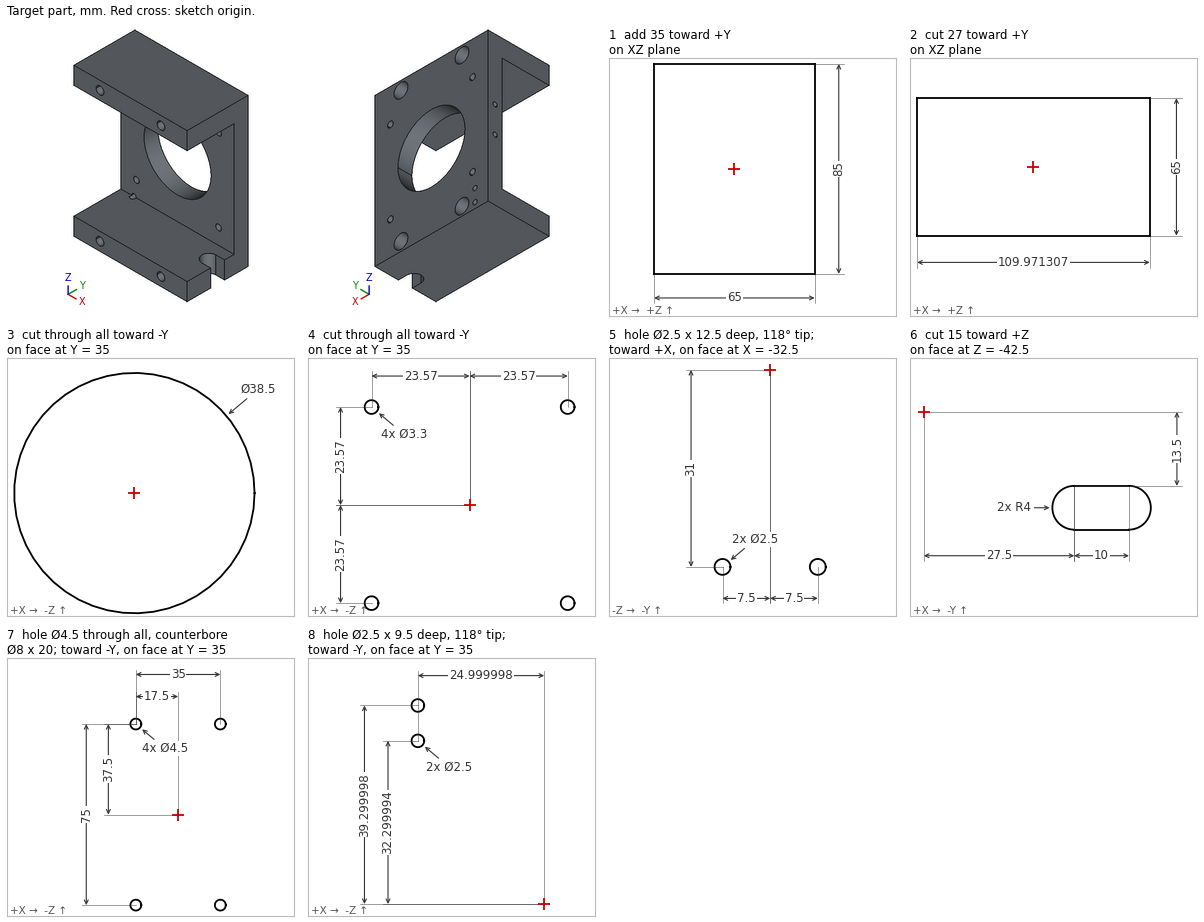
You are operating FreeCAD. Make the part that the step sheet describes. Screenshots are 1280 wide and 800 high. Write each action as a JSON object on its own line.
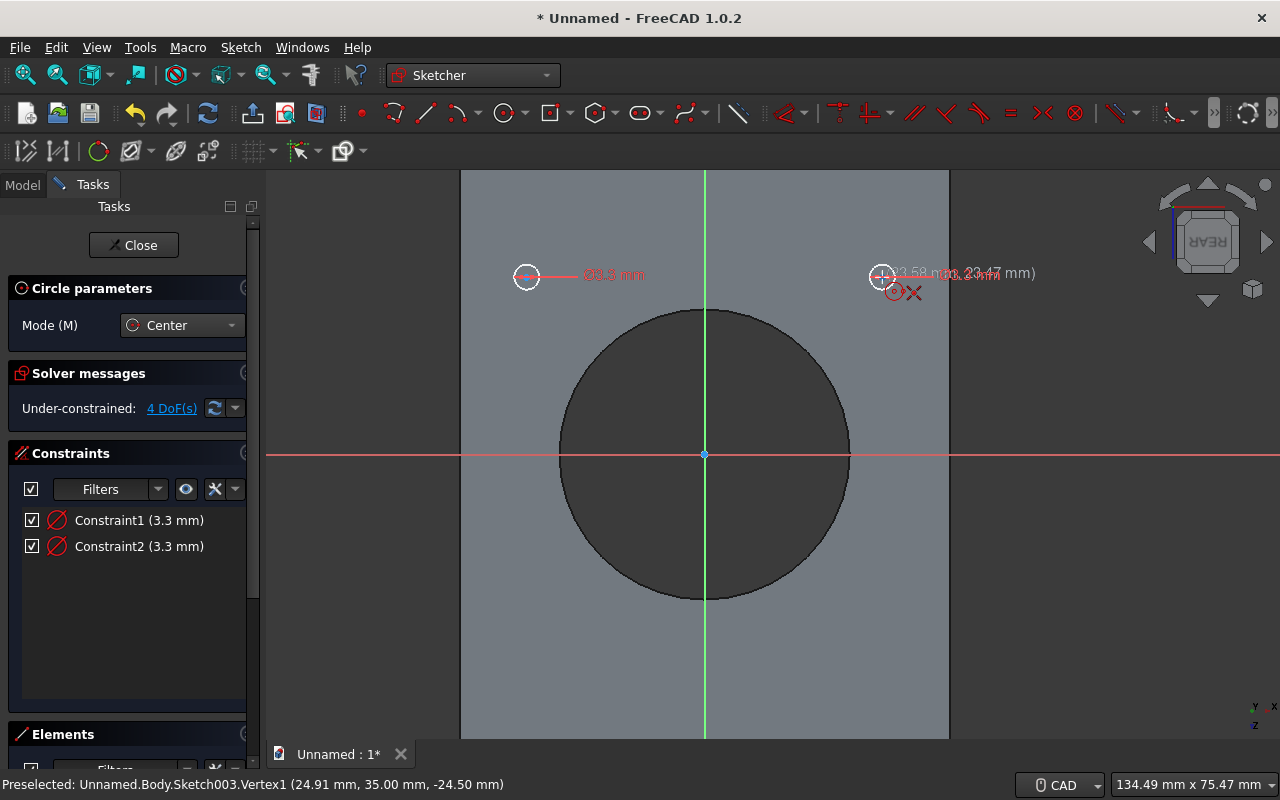
{"action": "scroll", "coordinate": [527, 632], "scroll_direction": "up", "scroll_amount": 4}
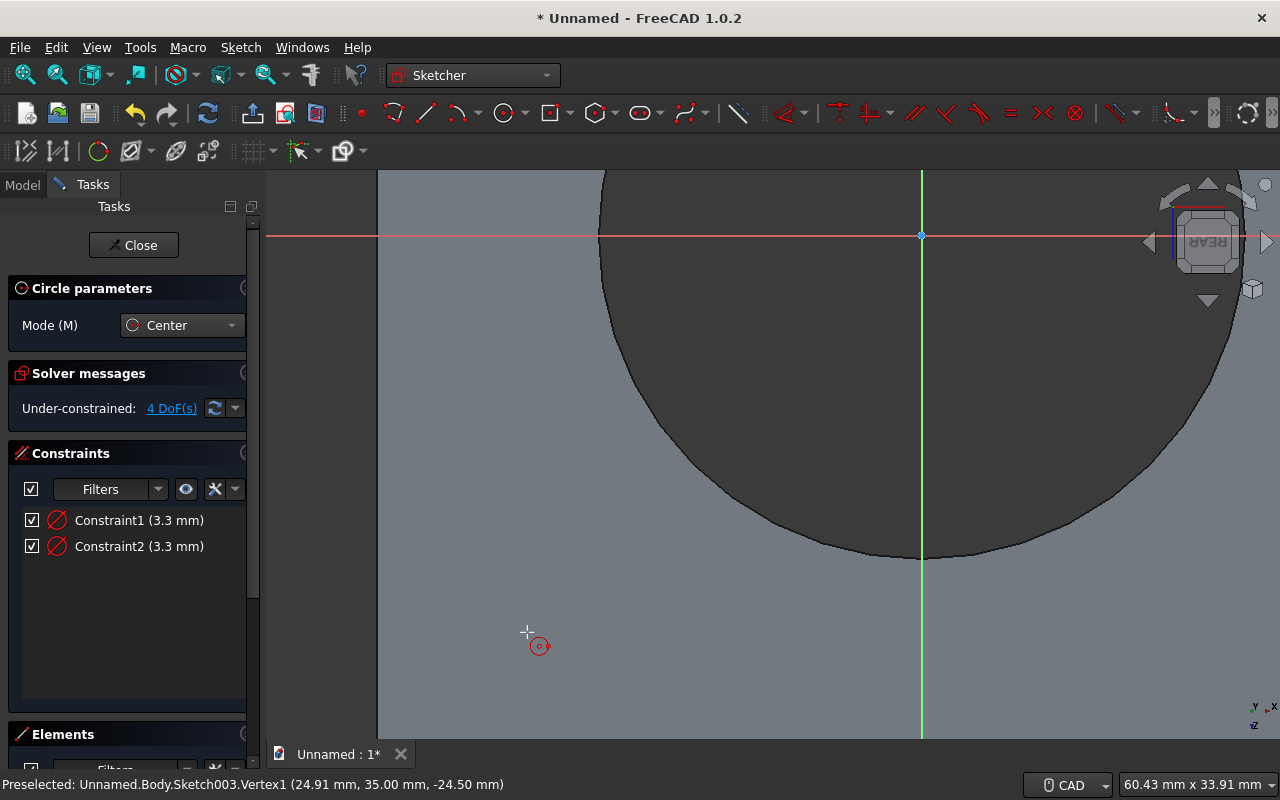
{"action": "left_click", "coordinate": [526, 631]}
{"action": "mouse_move", "coordinate": [546, 612]}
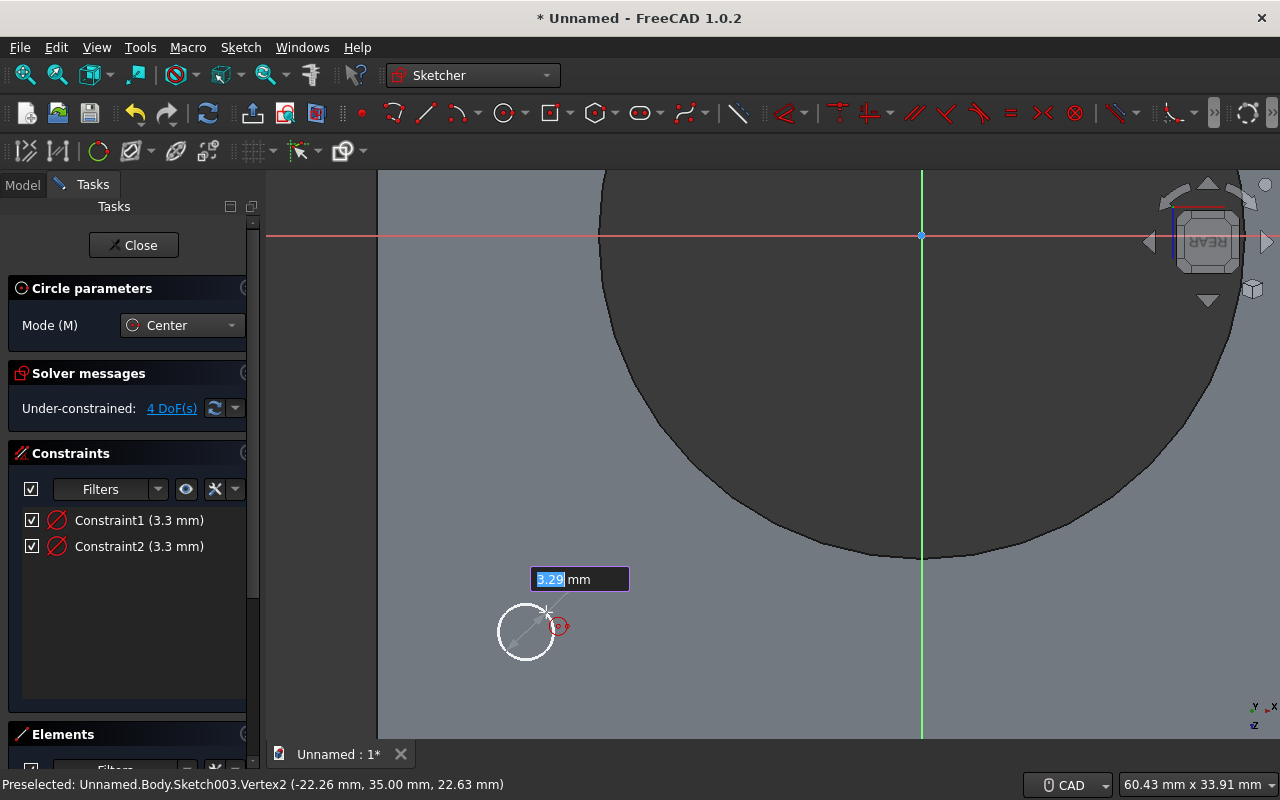
{"action": "type", "text": "3.3"}
{"action": "key", "text": "Return"}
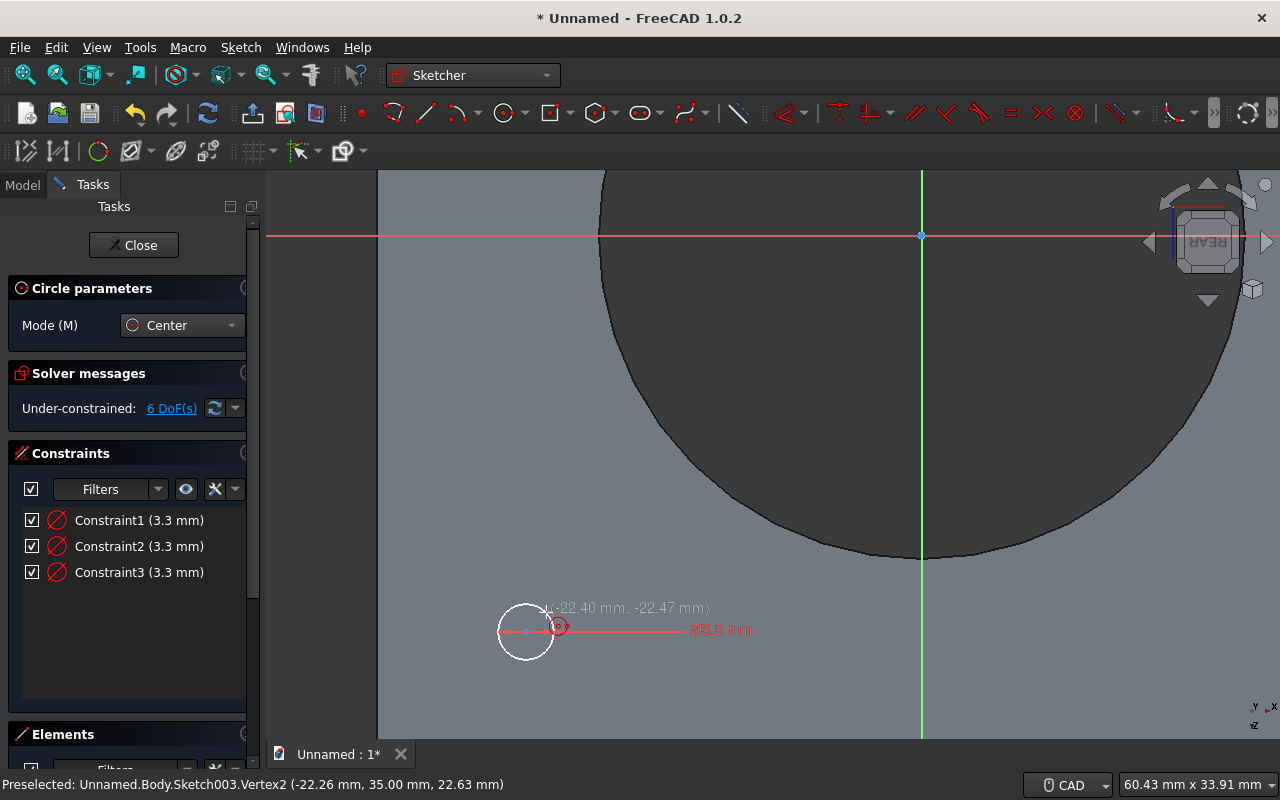
{"action": "scroll", "coordinate": [527, 633], "scroll_direction": "down", "scroll_amount": 4}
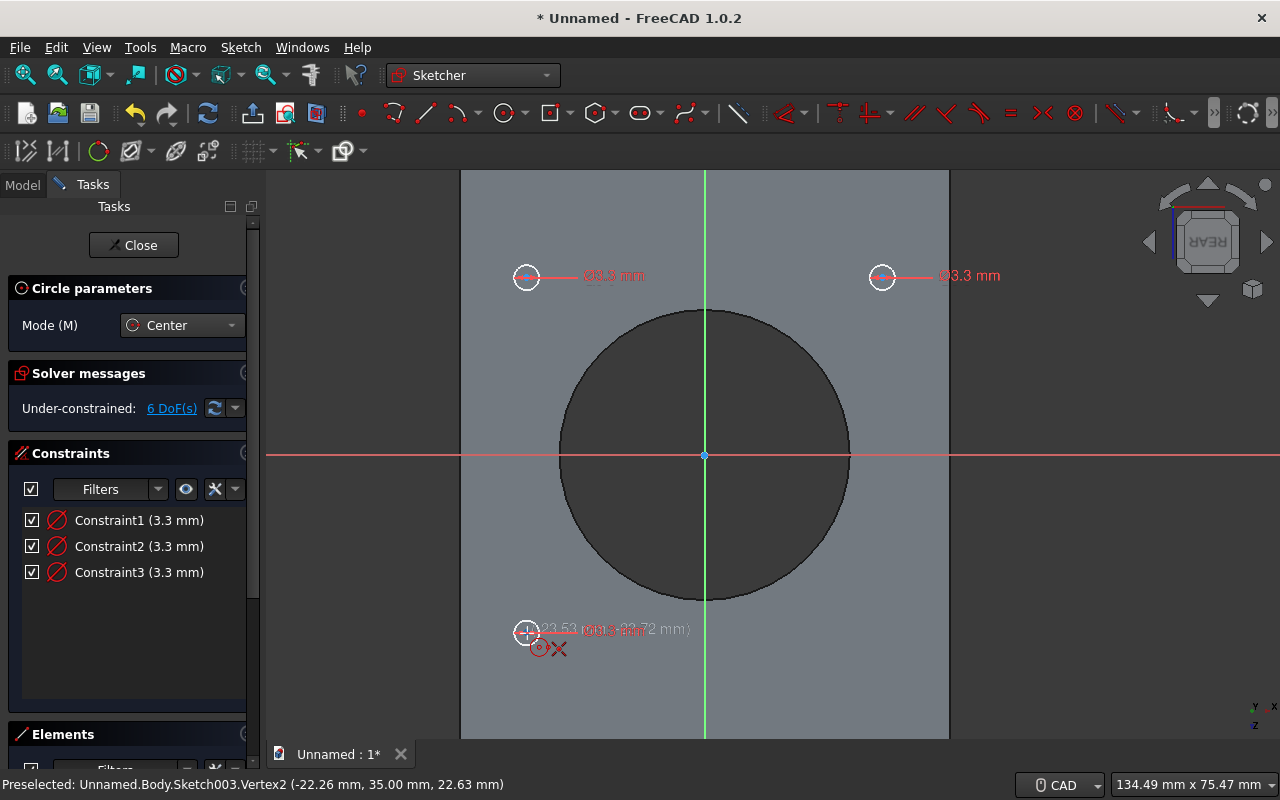
{"action": "scroll", "coordinate": [882, 633], "scroll_direction": "up", "scroll_amount": 4}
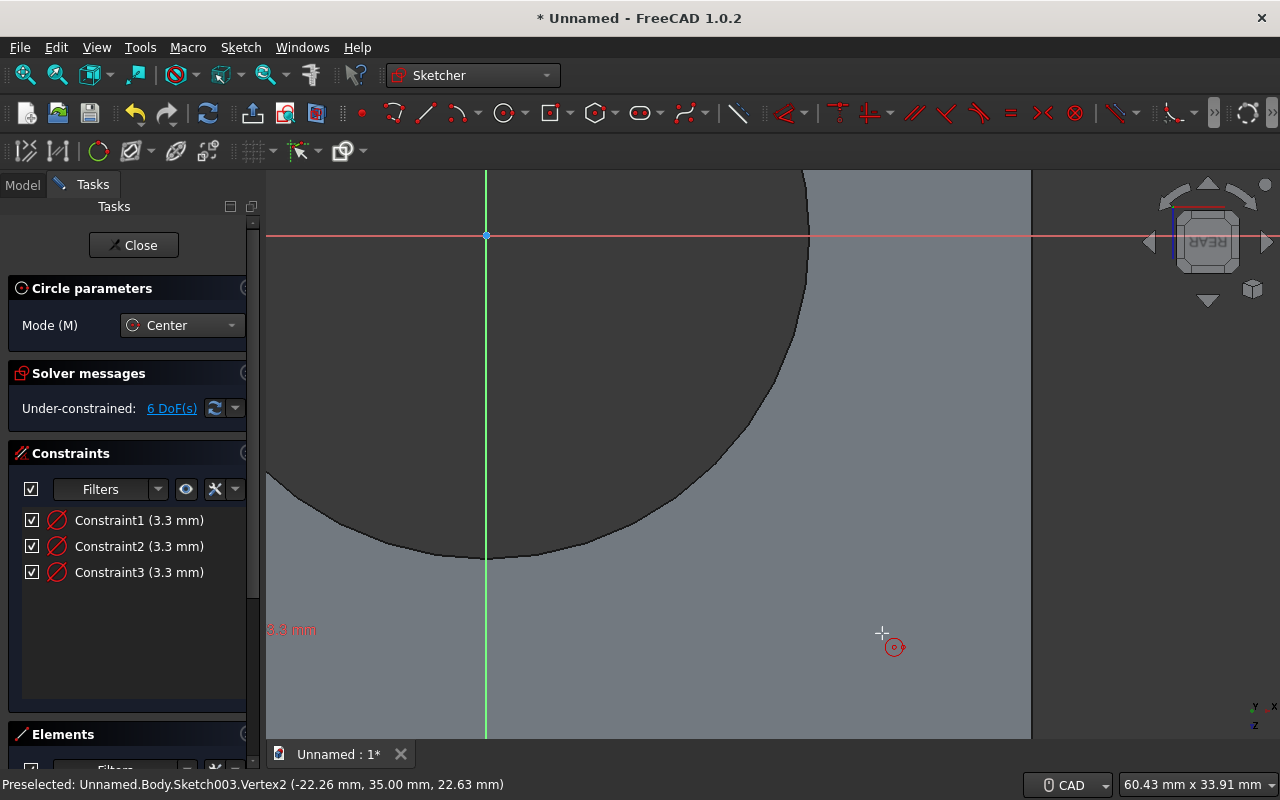
{"action": "left_click", "coordinate": [882, 631]}
{"action": "mouse_move", "coordinate": [901, 612]}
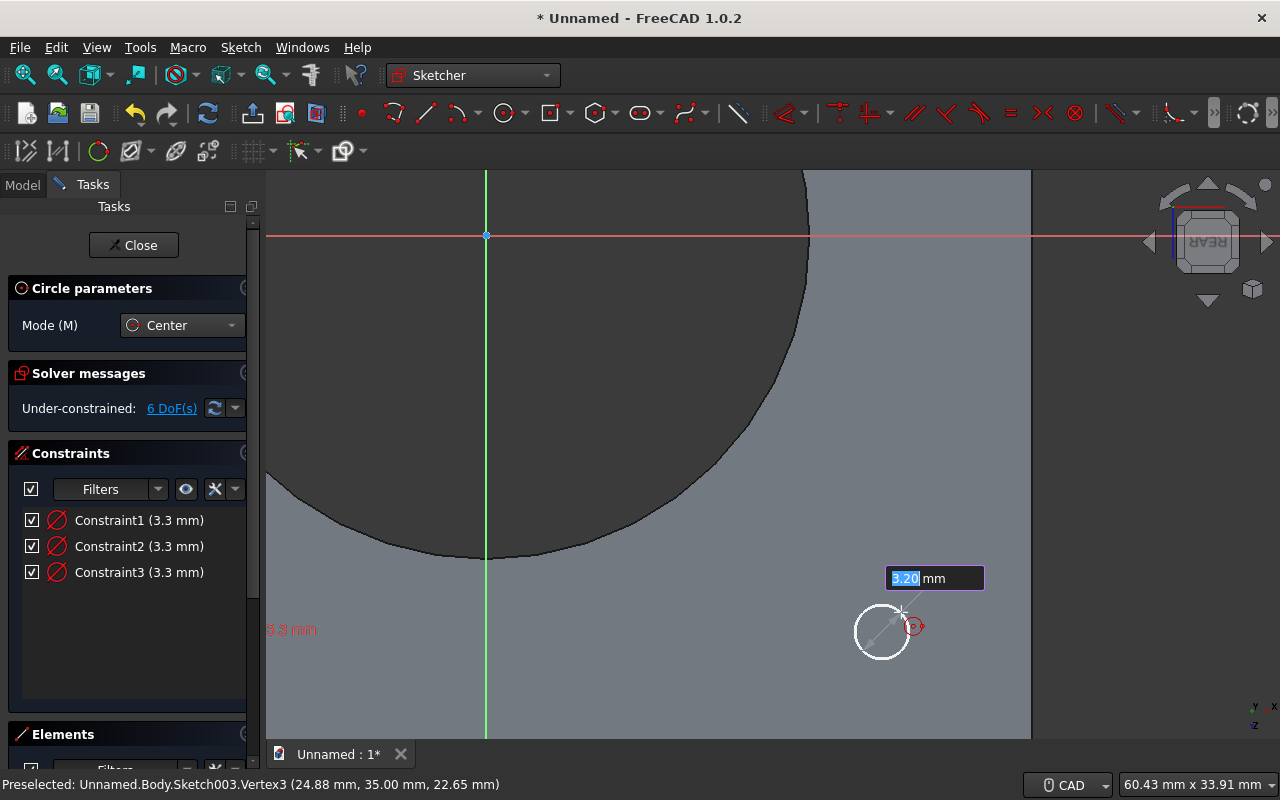
{"action": "type", "text": "3.3"}
{"action": "key", "text": "Return"}
{"action": "key", "text": "Escape"}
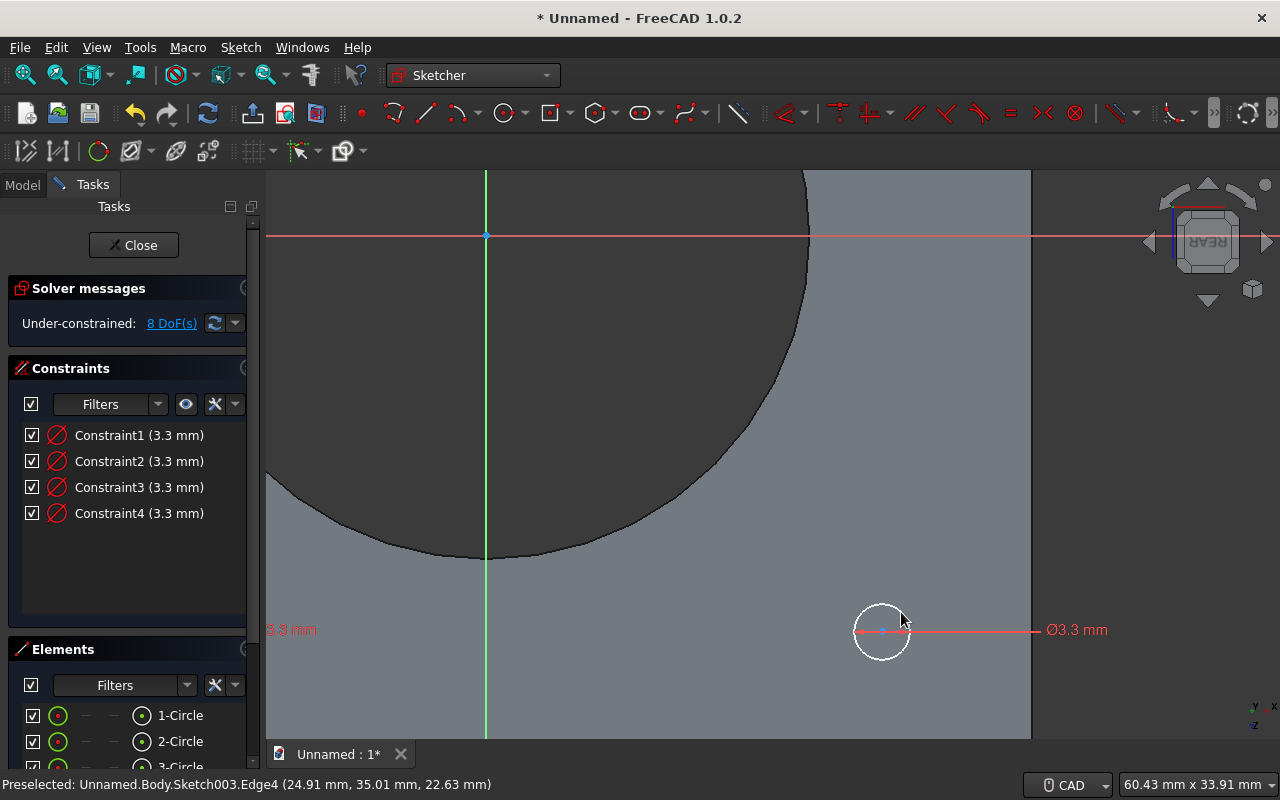
{"action": "scroll", "coordinate": [882, 633], "scroll_direction": "down", "scroll_amount": 4}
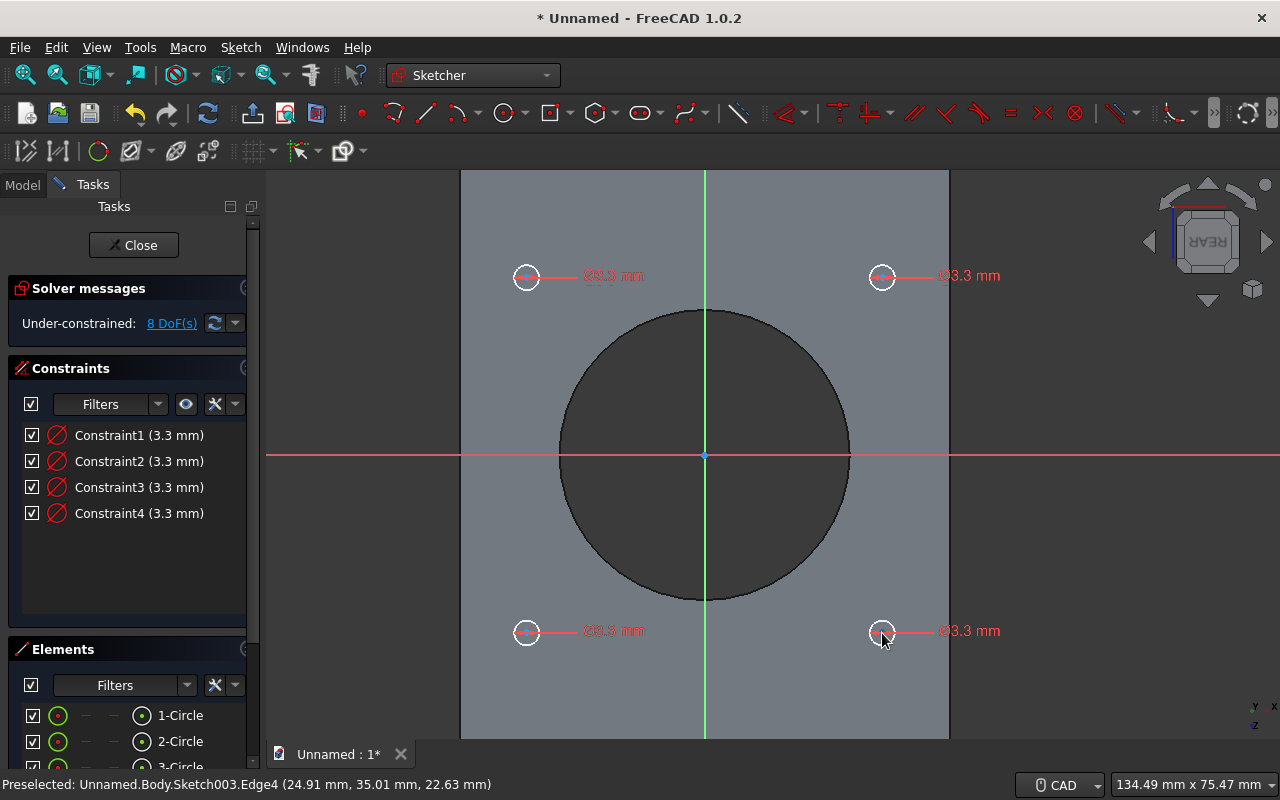
{"action": "left_click", "coordinate": [527, 278]}